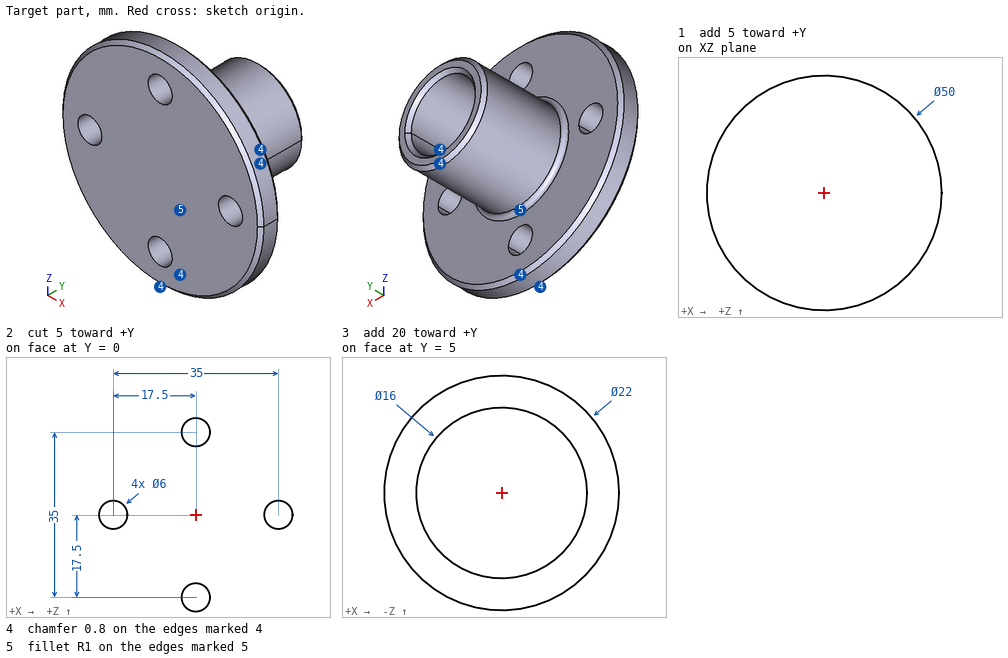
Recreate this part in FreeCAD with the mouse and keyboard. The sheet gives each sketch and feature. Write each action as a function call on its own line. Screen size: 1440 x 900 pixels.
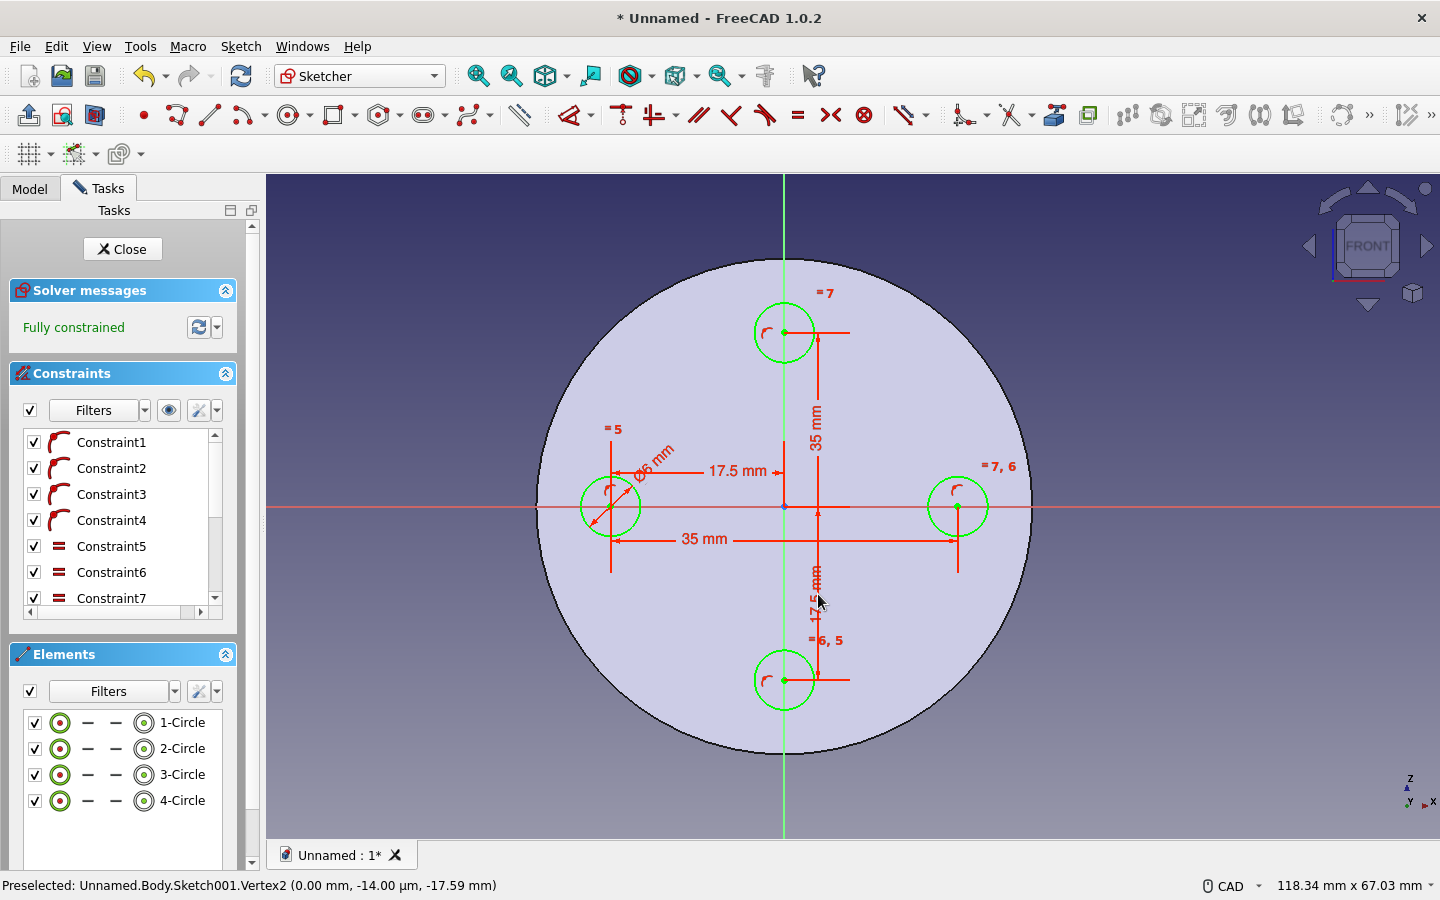
click(123, 249)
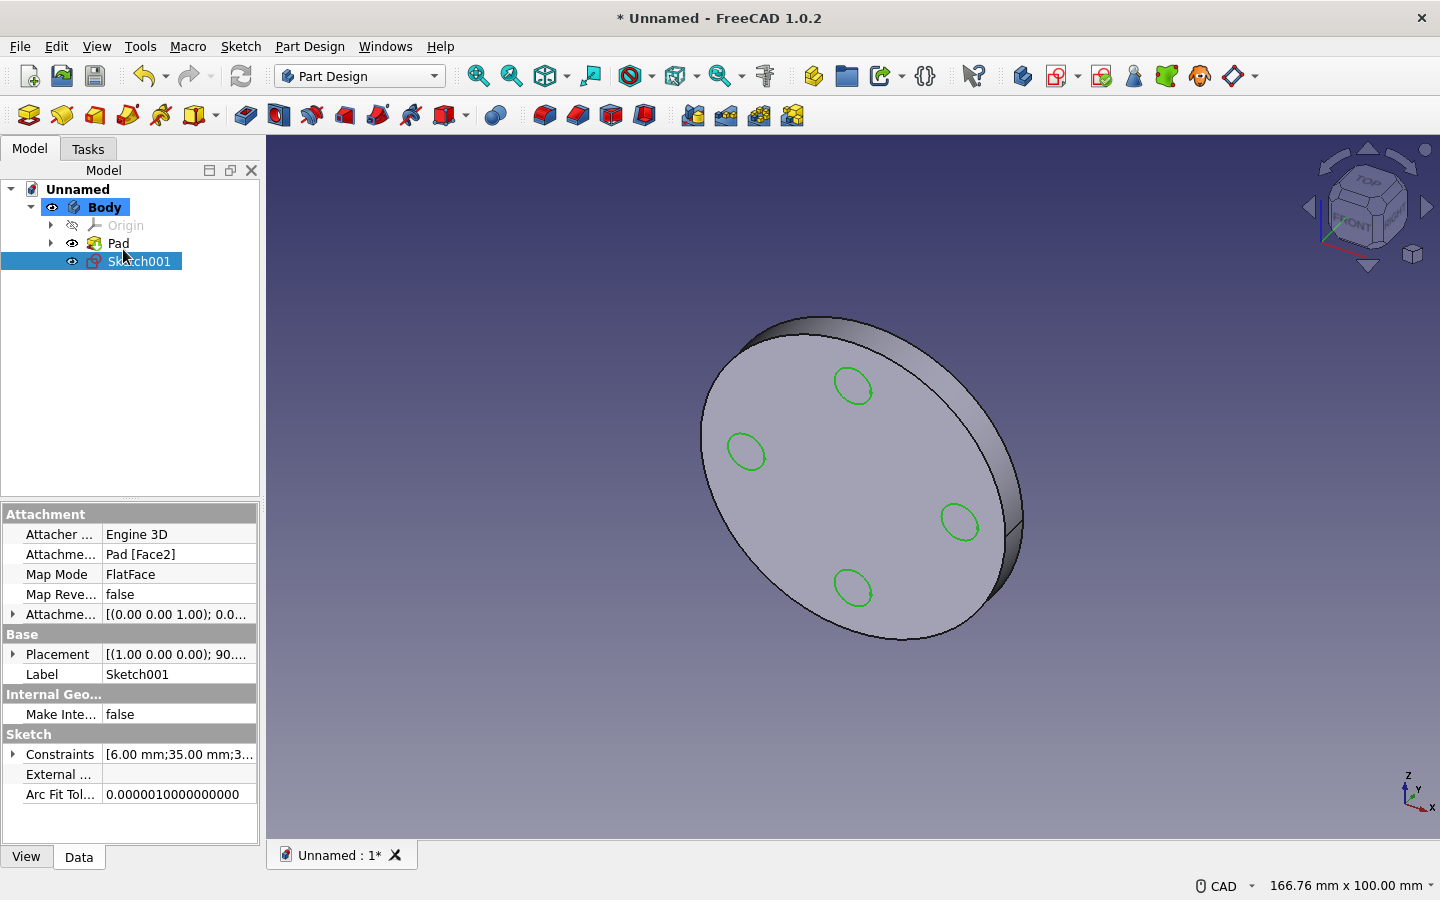
click(246, 116)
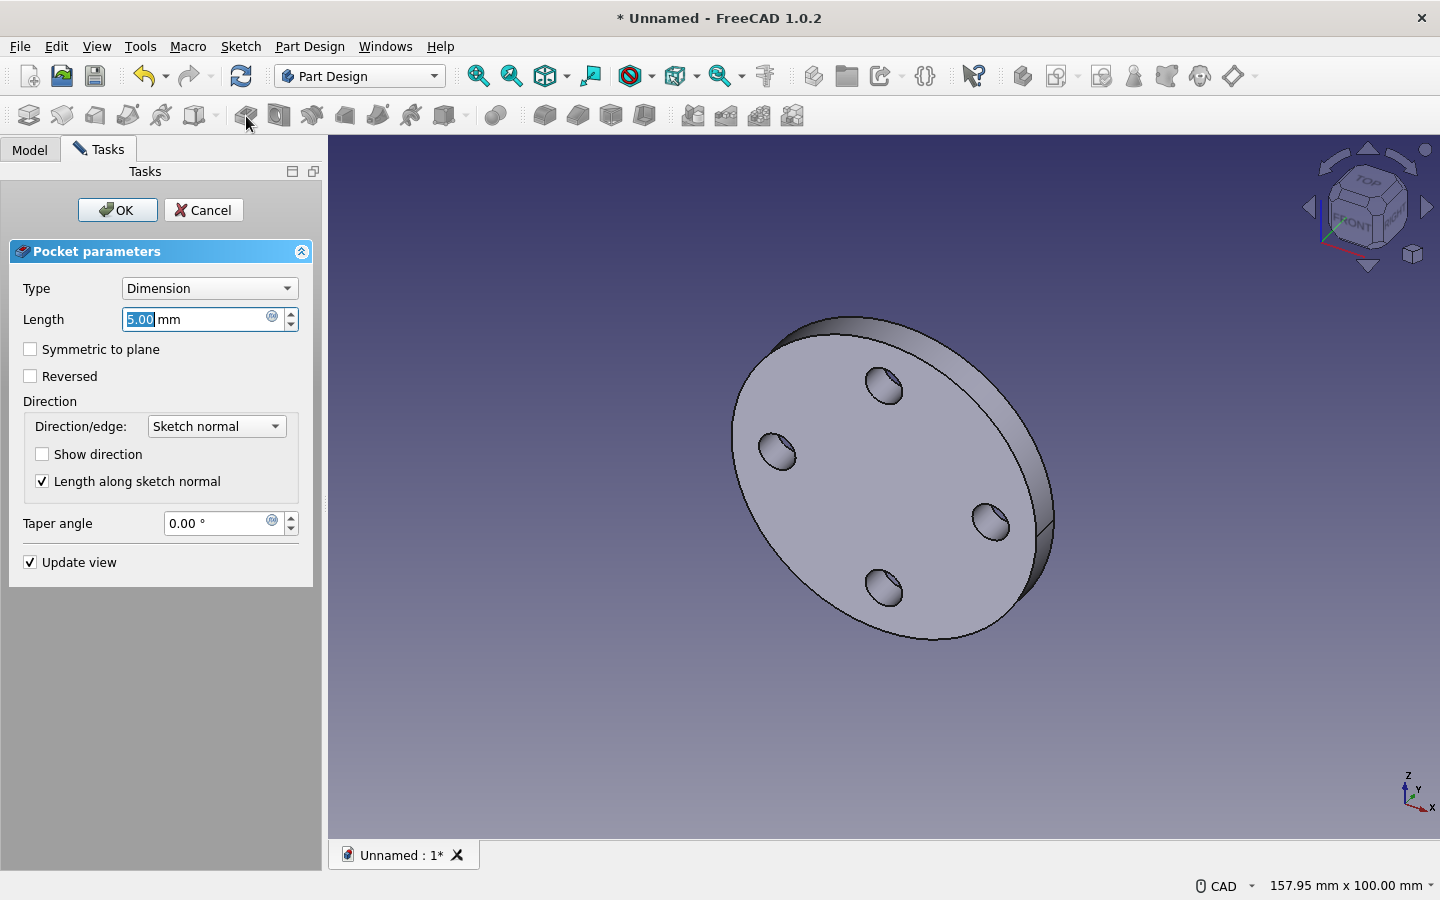
text(5)
key(Tab)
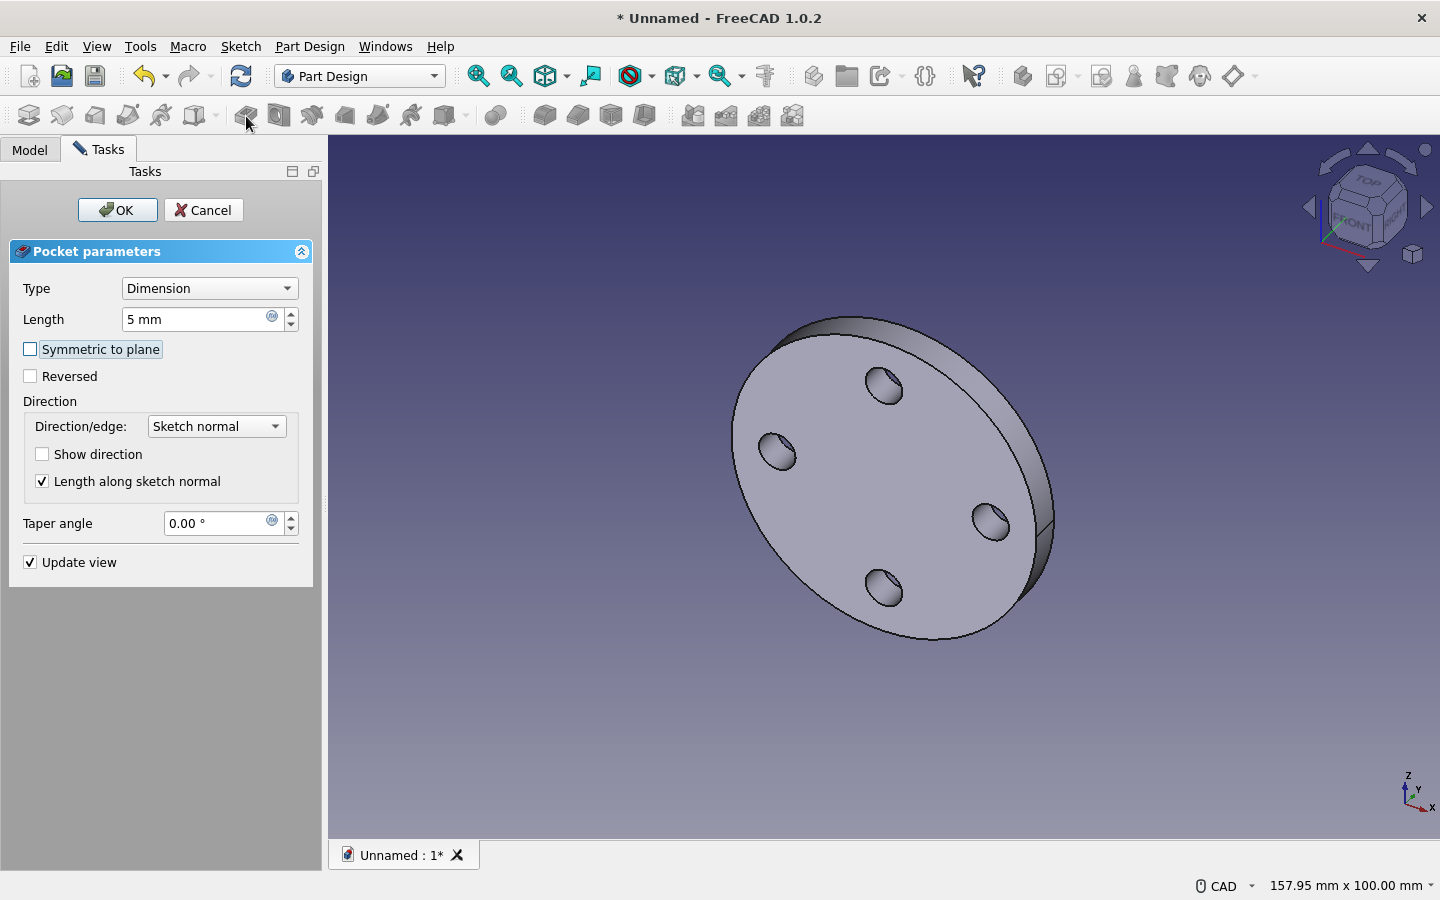
click(118, 210)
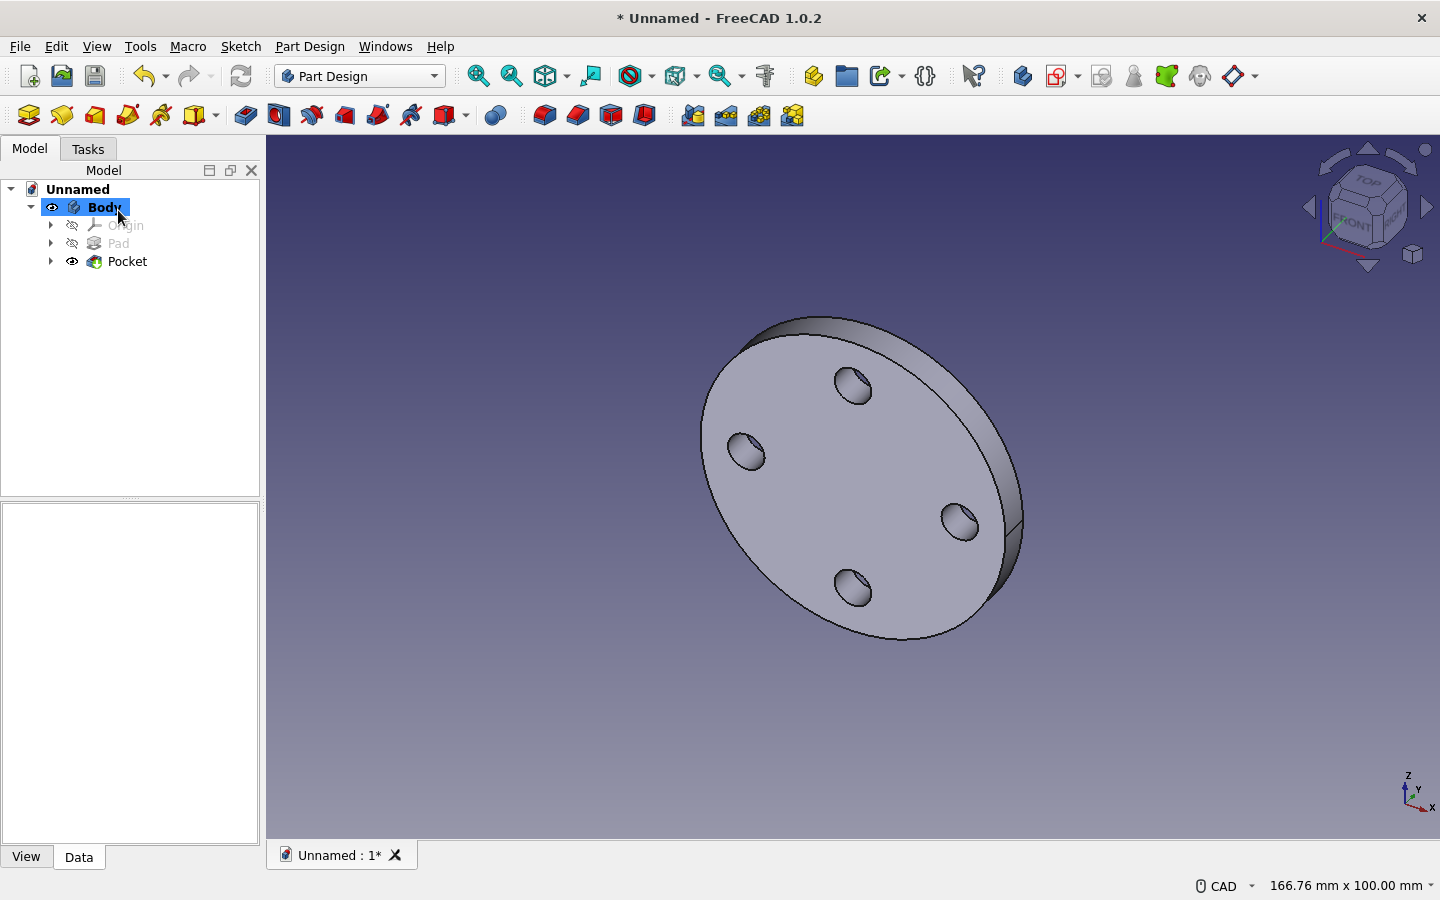
key(4)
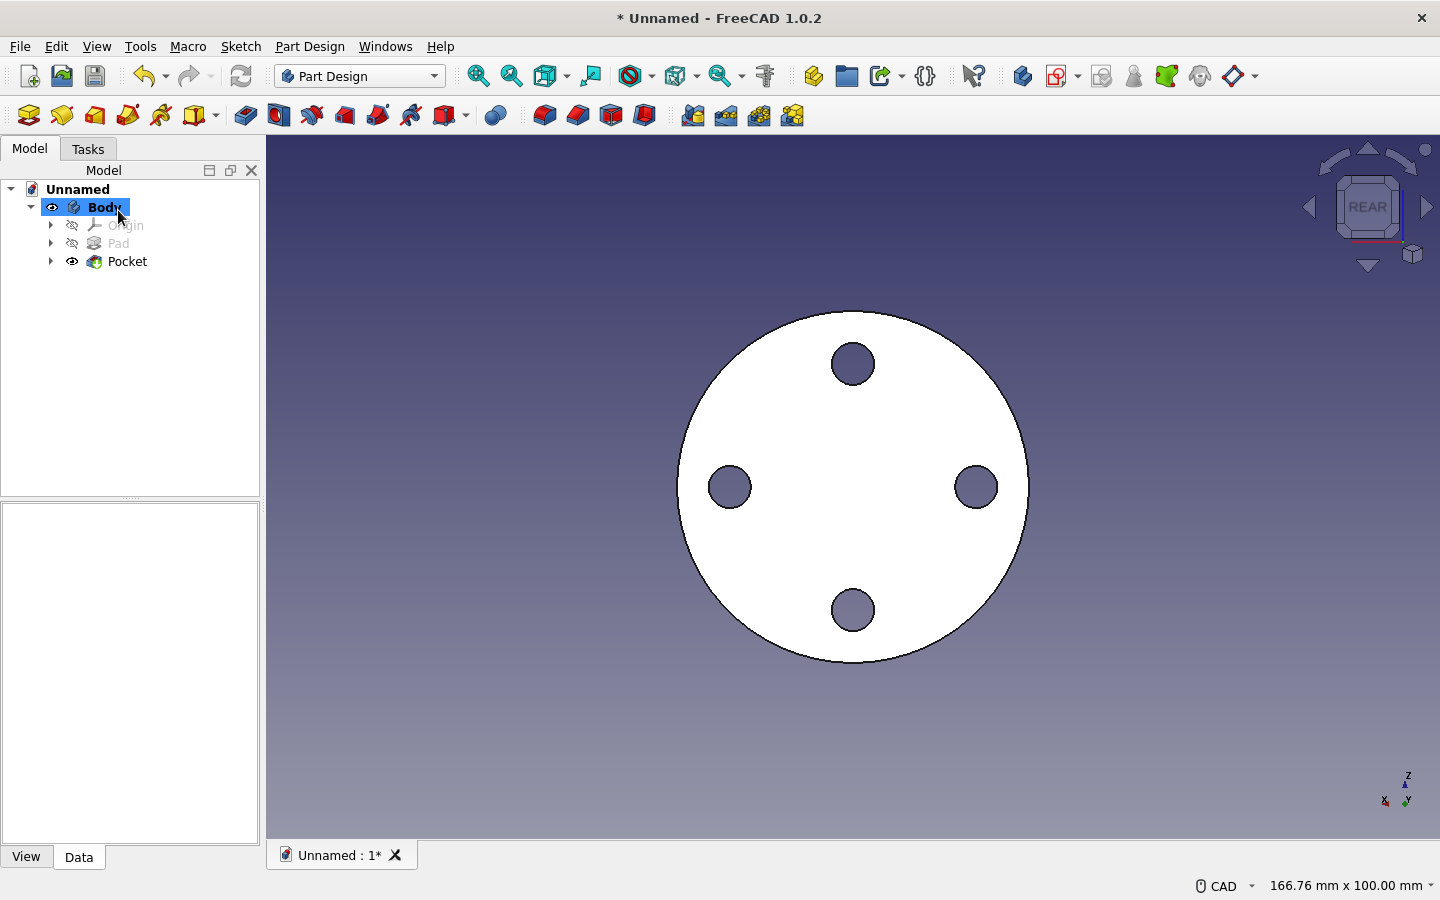
click(853, 486)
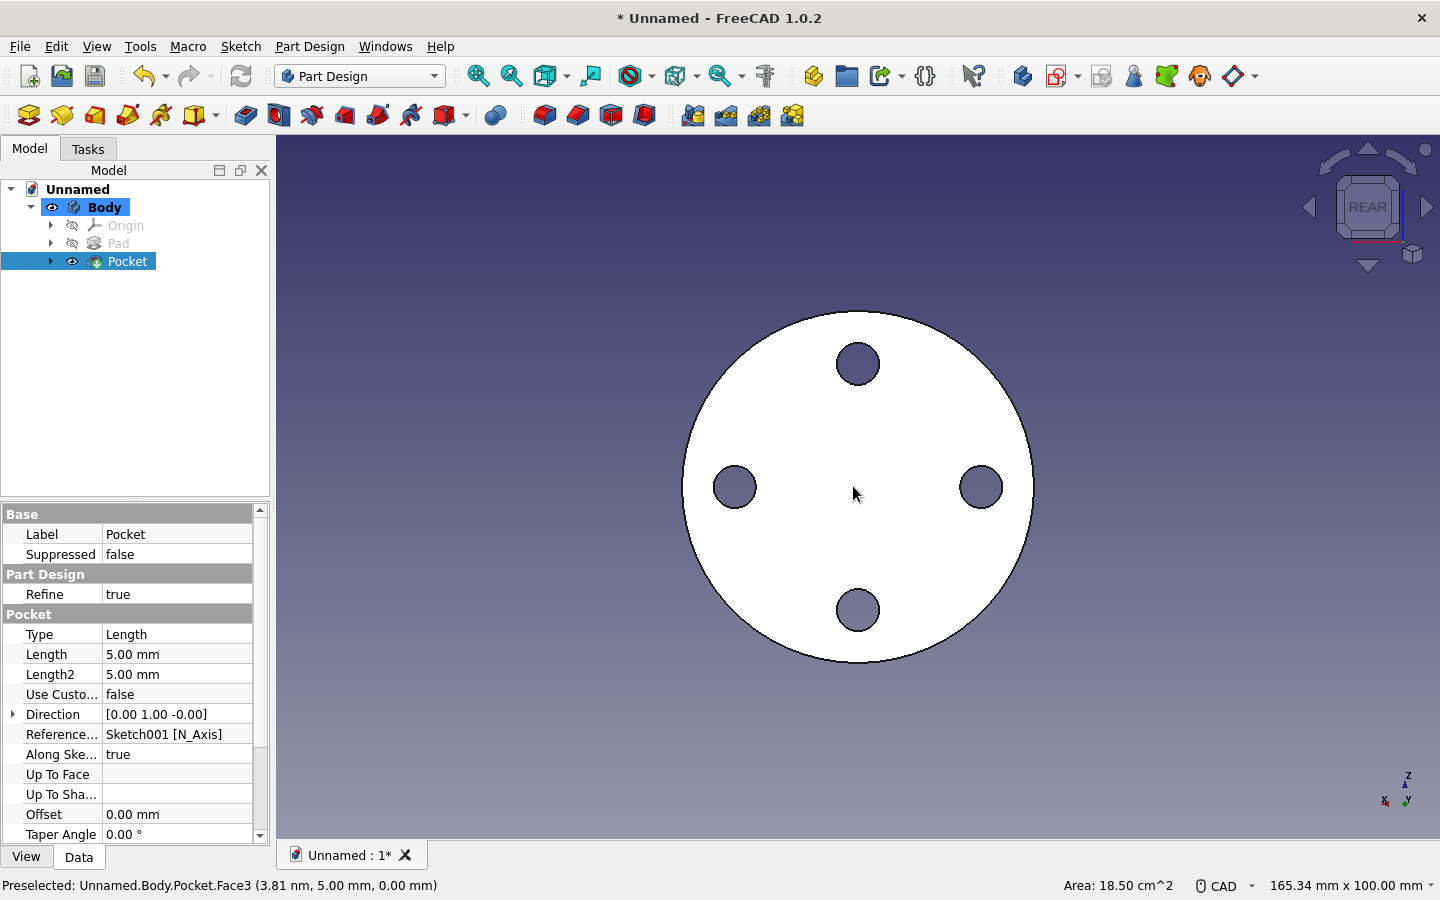
click(1056, 76)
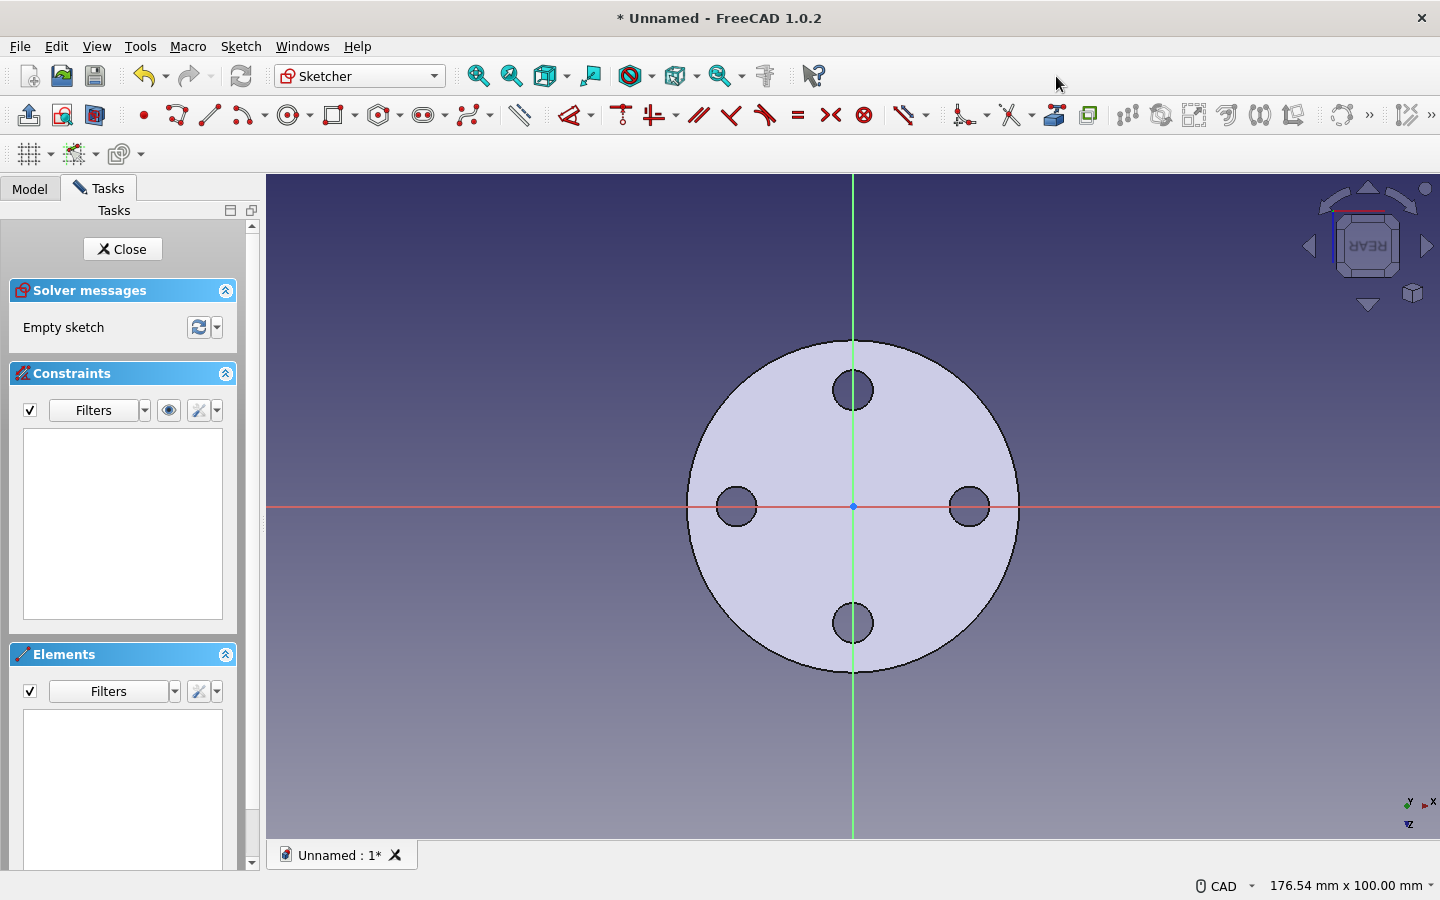
scroll(893, 507, up, 5)